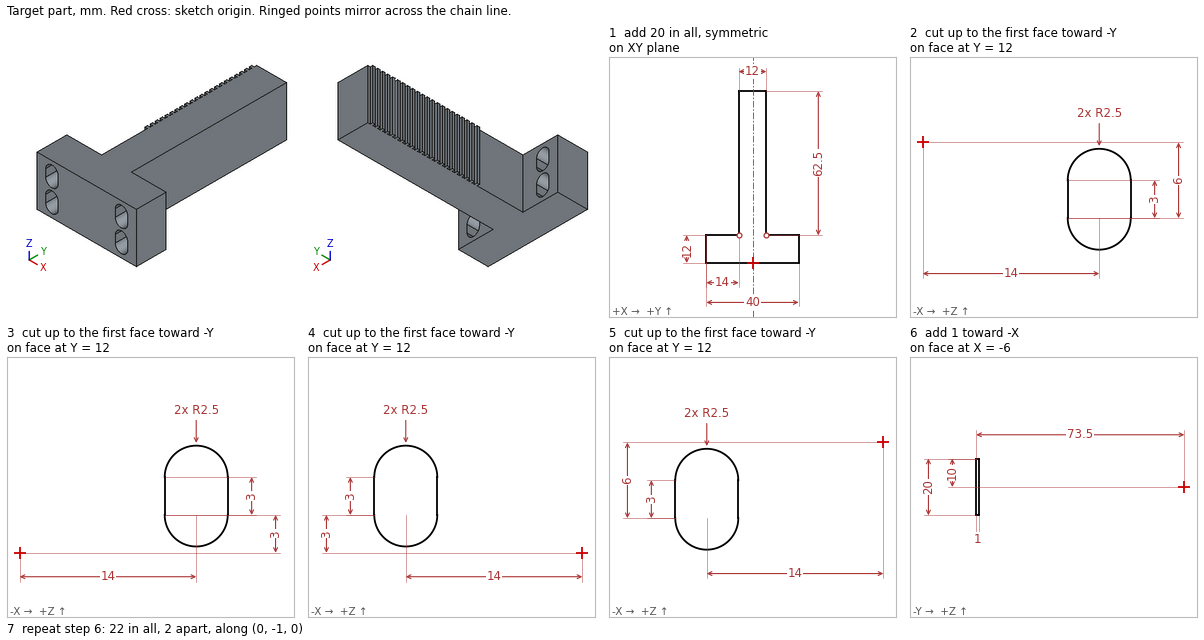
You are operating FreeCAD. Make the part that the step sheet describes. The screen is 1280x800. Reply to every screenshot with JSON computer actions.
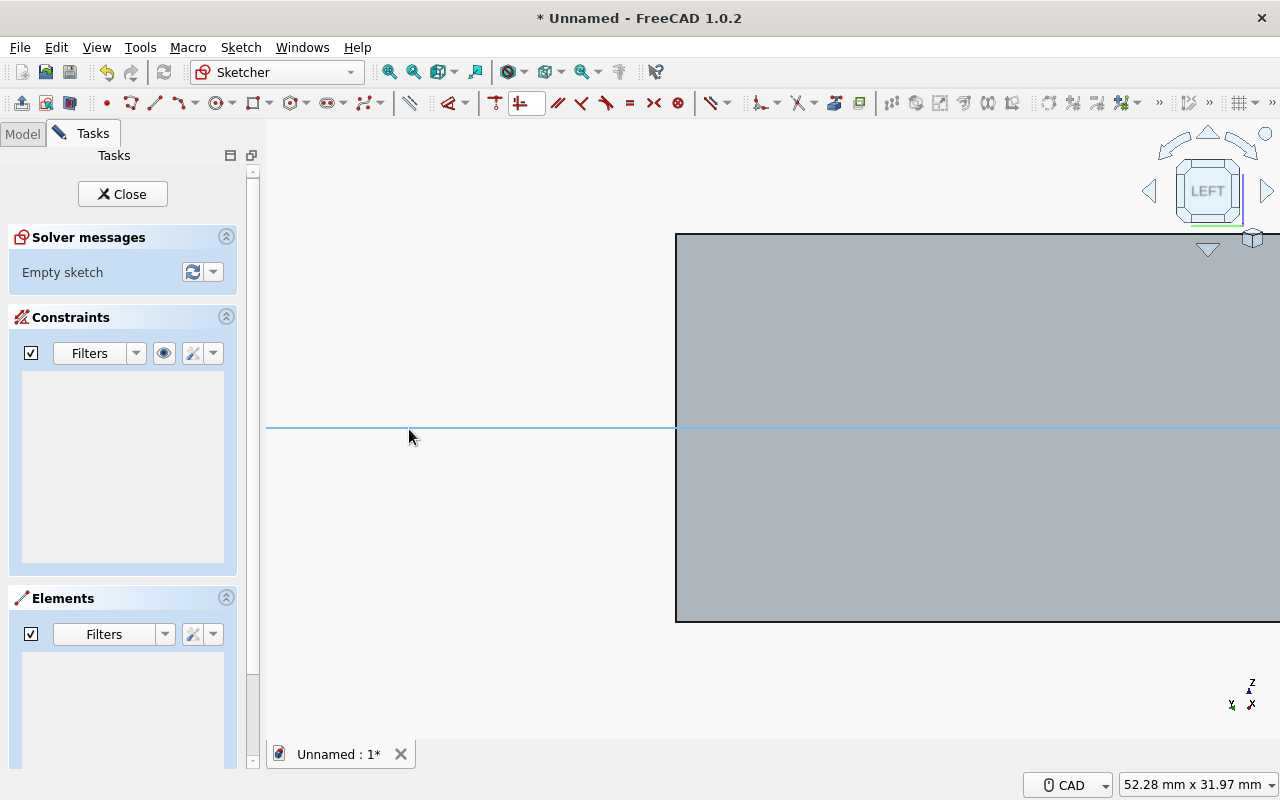
{"action": "left_click", "coordinate": [254, 104]}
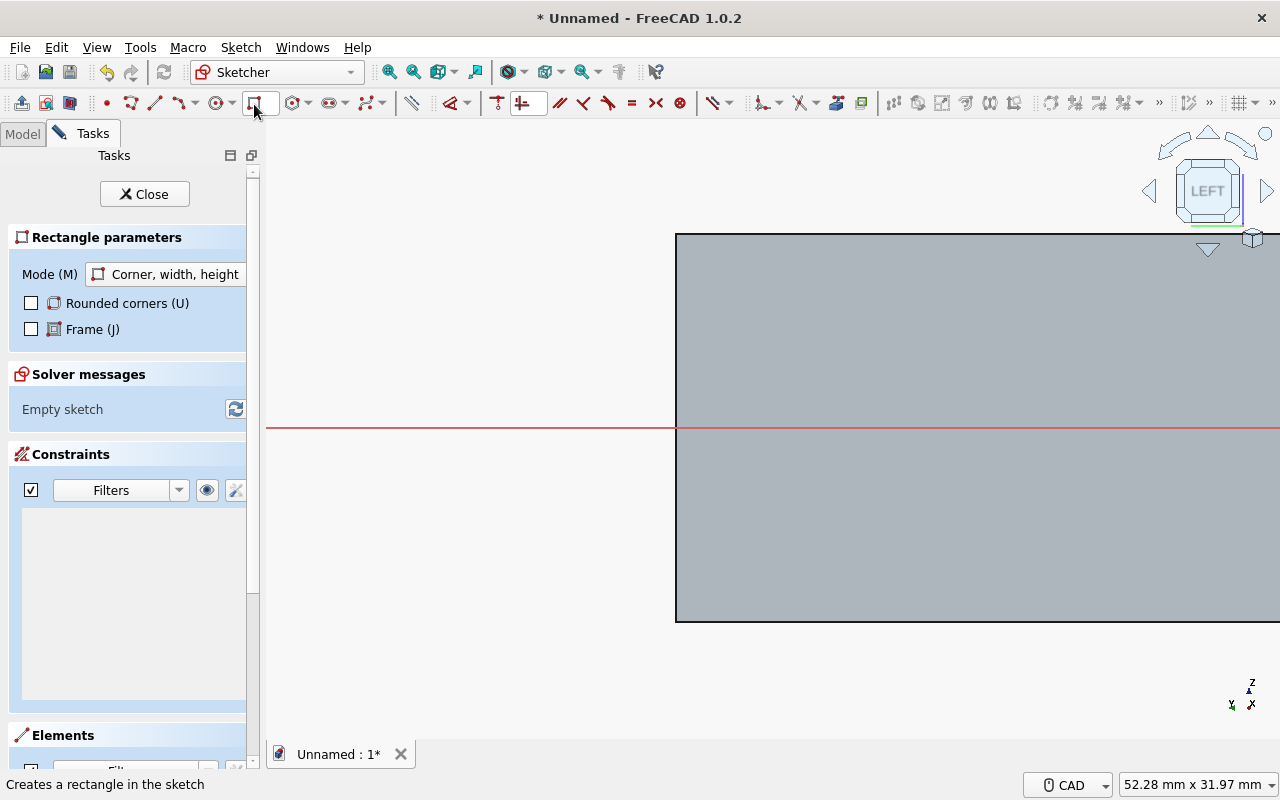
{"action": "left_click", "coordinate": [695, 234]}
{"action": "left_click", "coordinate": [715, 622]}
{"action": "key", "text": "Escape"}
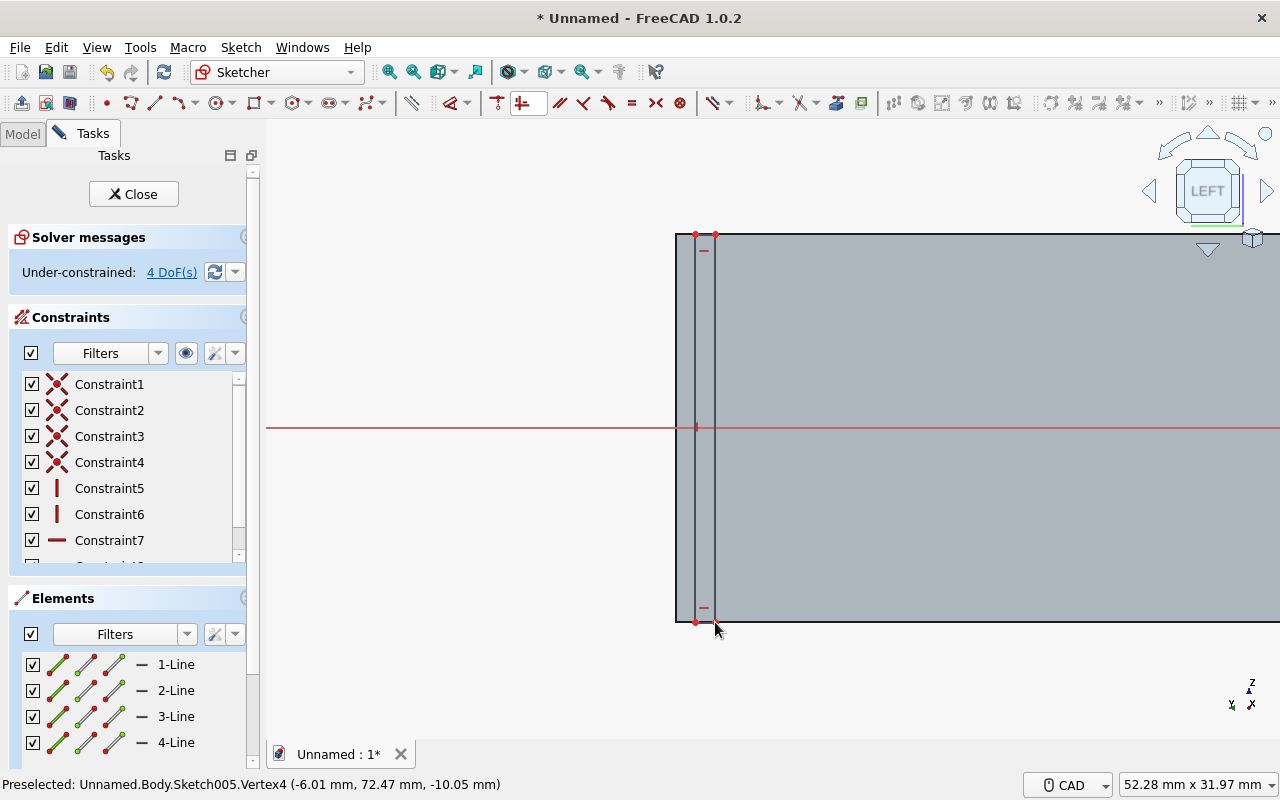
{"action": "left_click", "coordinate": [450, 104]}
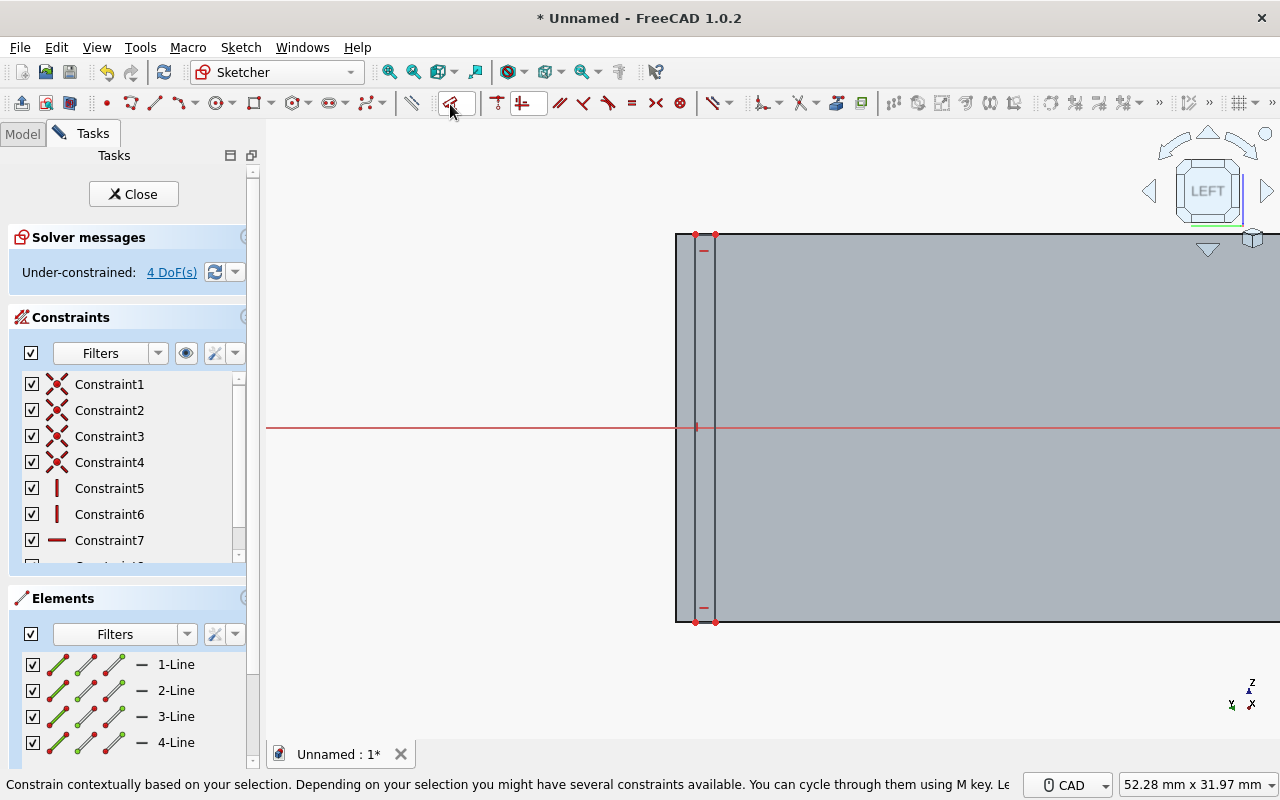
{"action": "scroll", "coordinate": [705, 623], "scroll_direction": "up", "scroll_amount": 4}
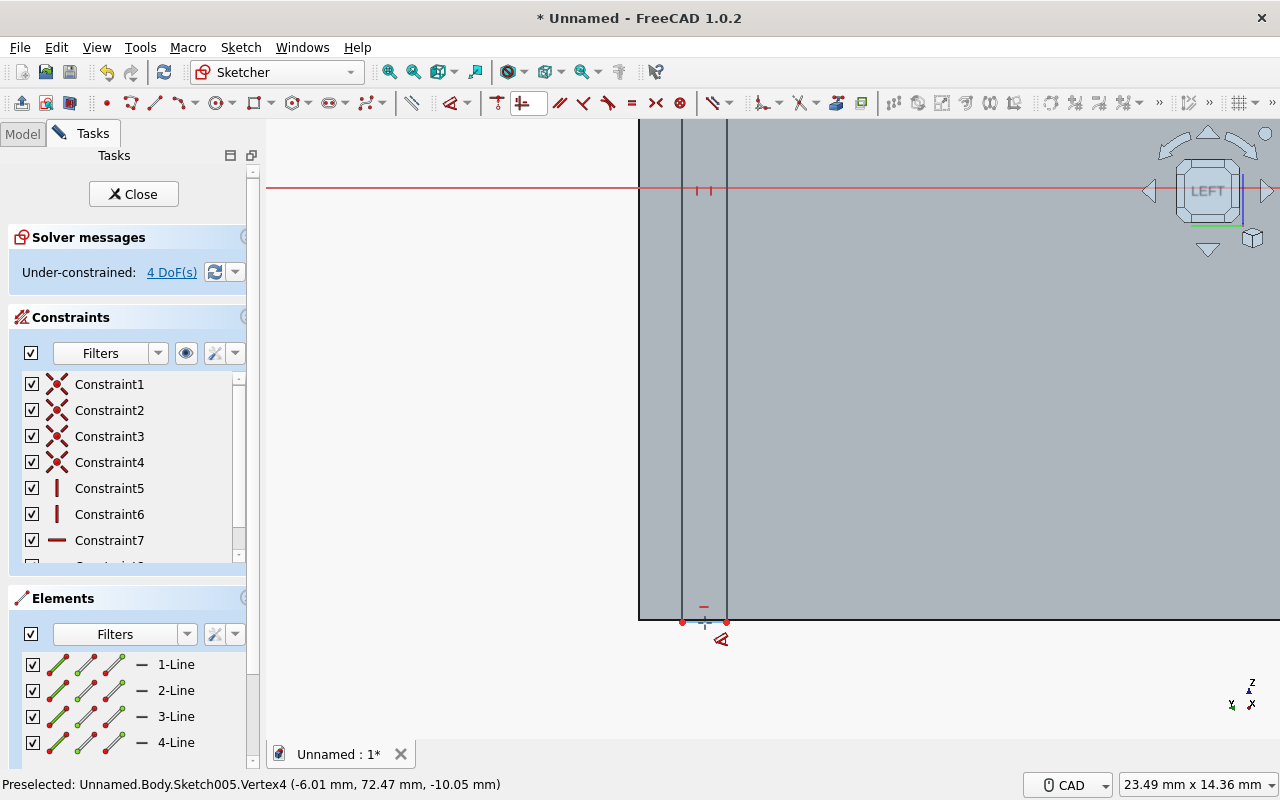
{"action": "left_click", "coordinate": [704, 622]}
{"action": "left_click", "coordinate": [704, 656]}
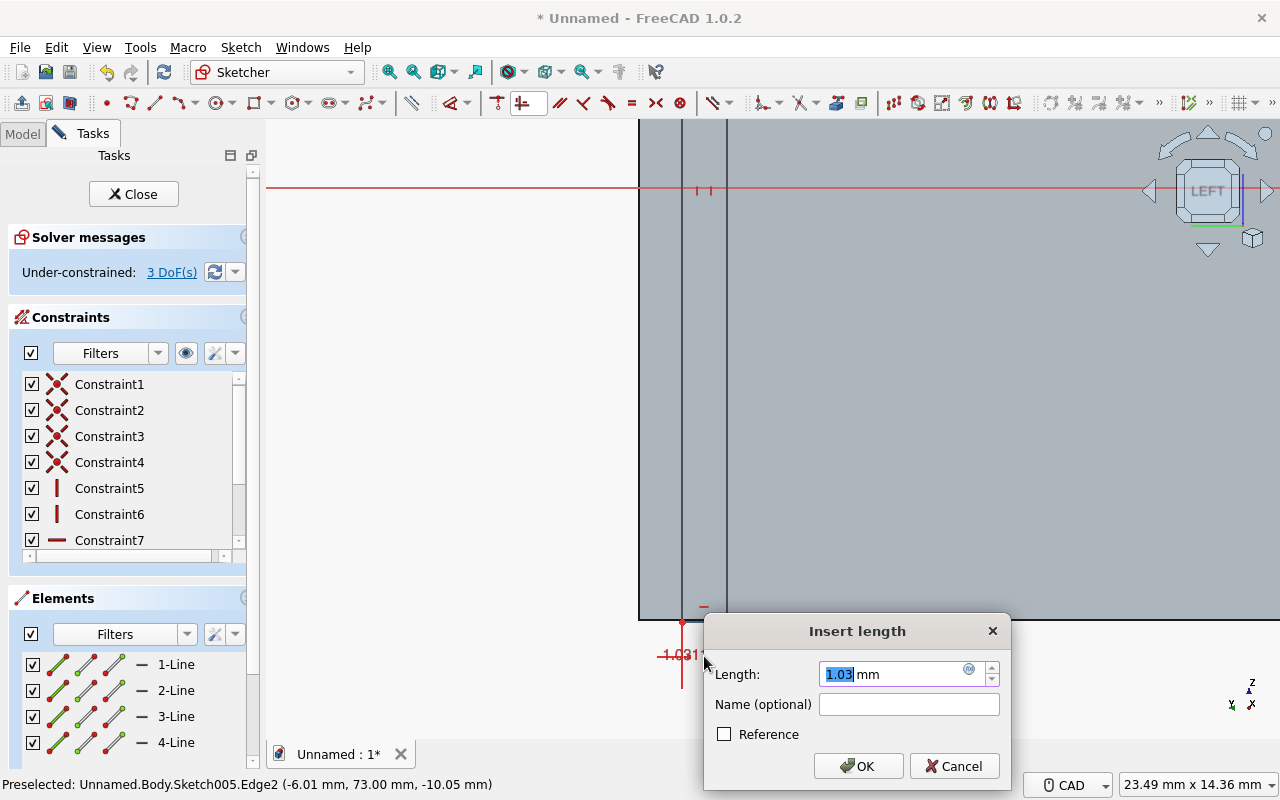
{"action": "type", "text": "1"}
{"action": "key", "text": "Return"}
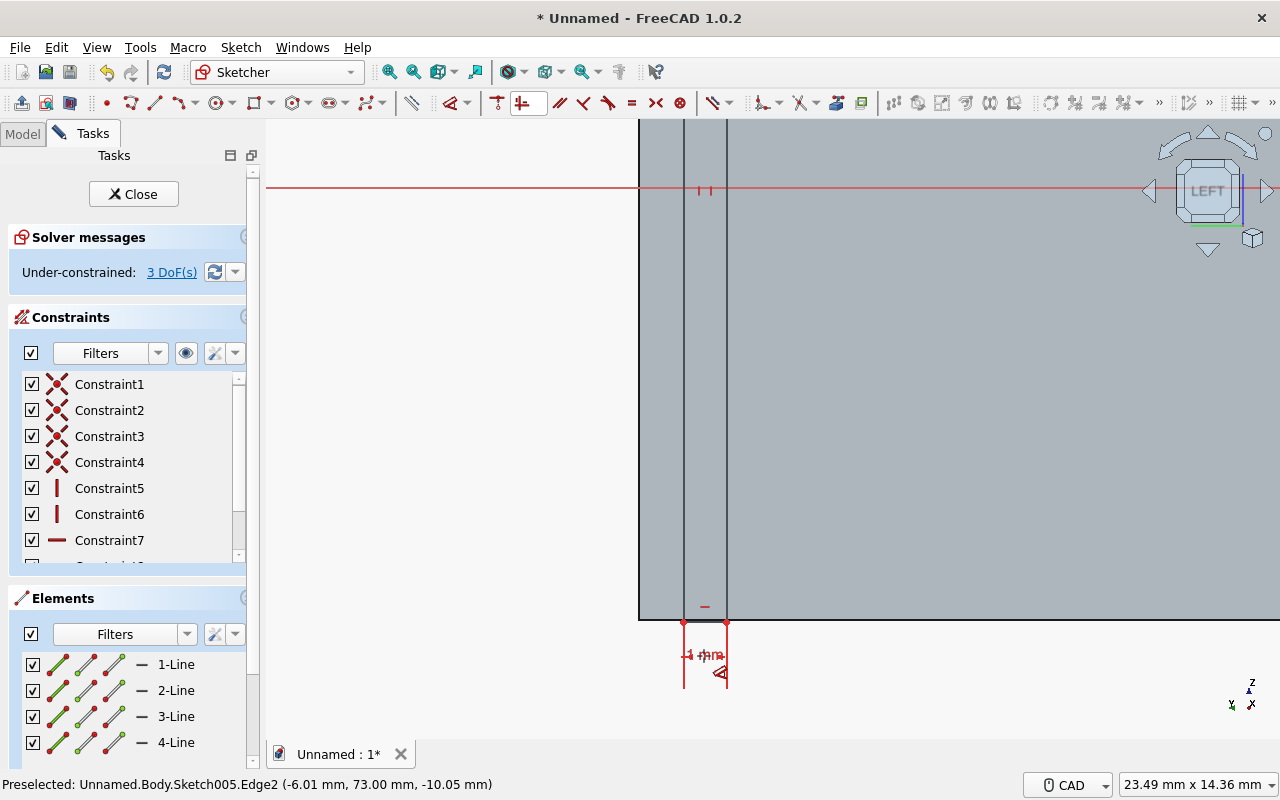
{"action": "left_click", "coordinate": [684, 363]}
{"action": "left_click", "coordinate": [650, 385]}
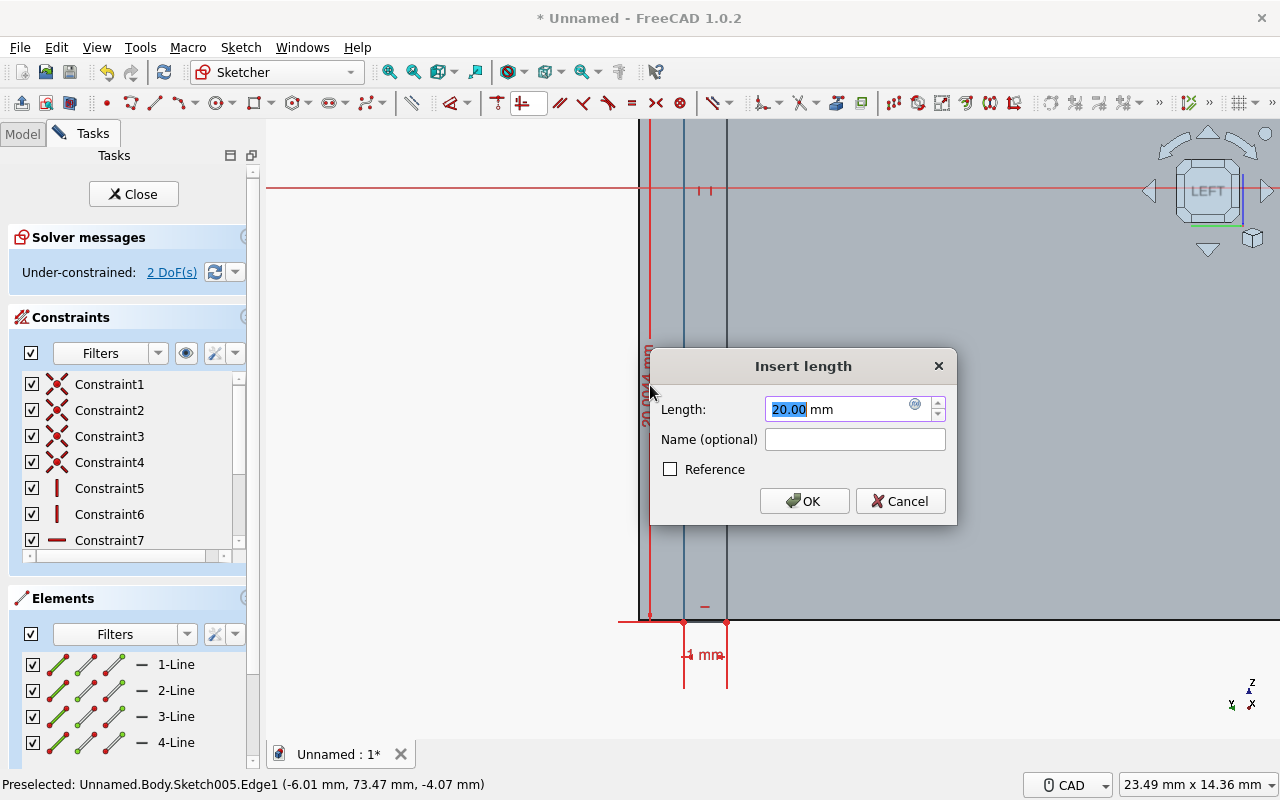
{"action": "type", "text": "20"}
{"action": "key", "text": "Return"}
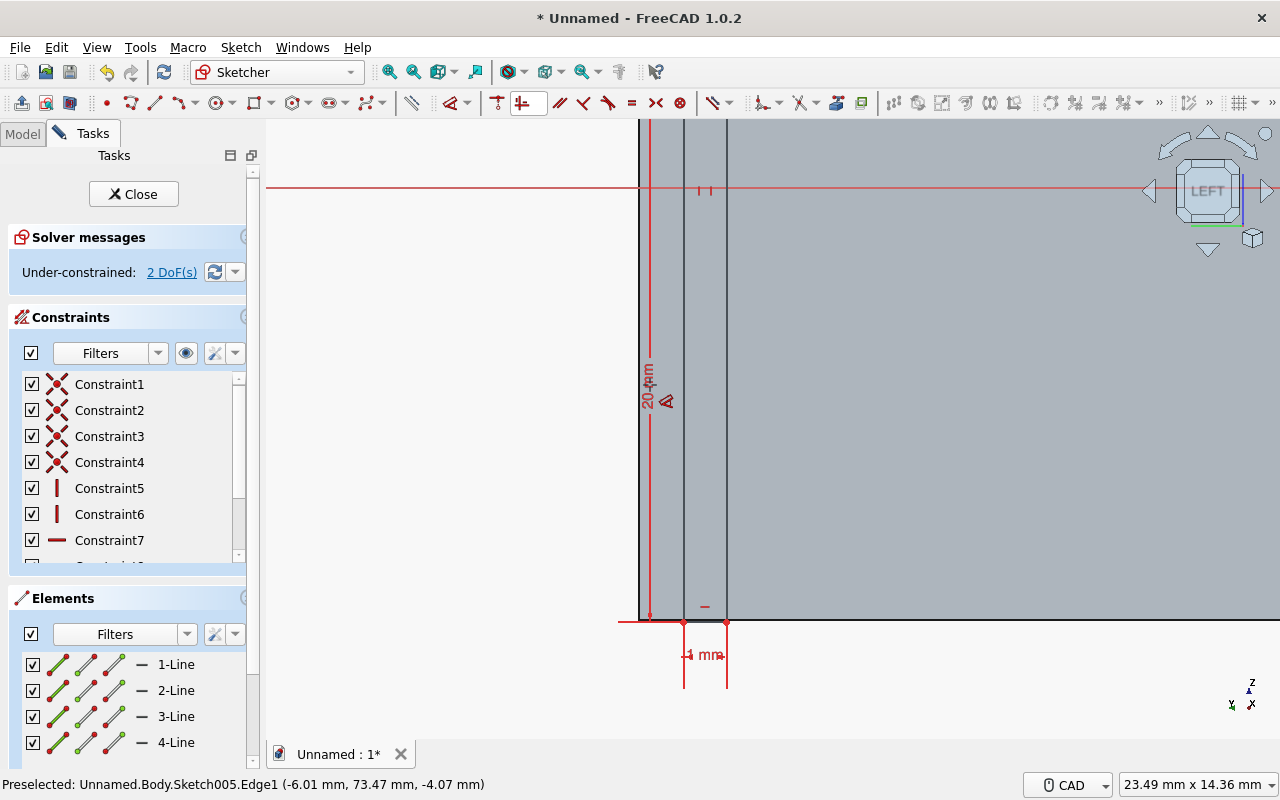
{"action": "scroll", "coordinate": [705, 625], "scroll_direction": "down", "scroll_amount": 4}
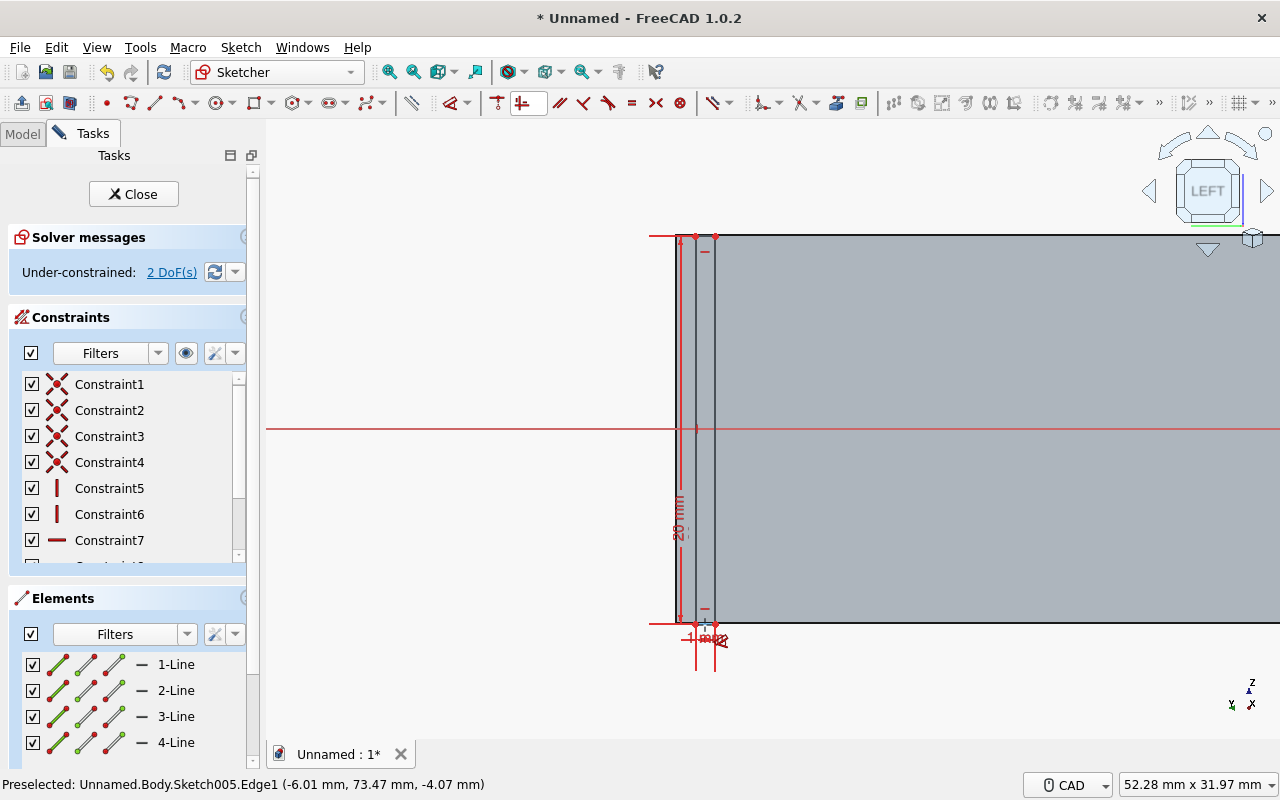
{"action": "left_click", "coordinate": [696, 236]}
{"action": "left_click", "coordinate": [662, 333]}